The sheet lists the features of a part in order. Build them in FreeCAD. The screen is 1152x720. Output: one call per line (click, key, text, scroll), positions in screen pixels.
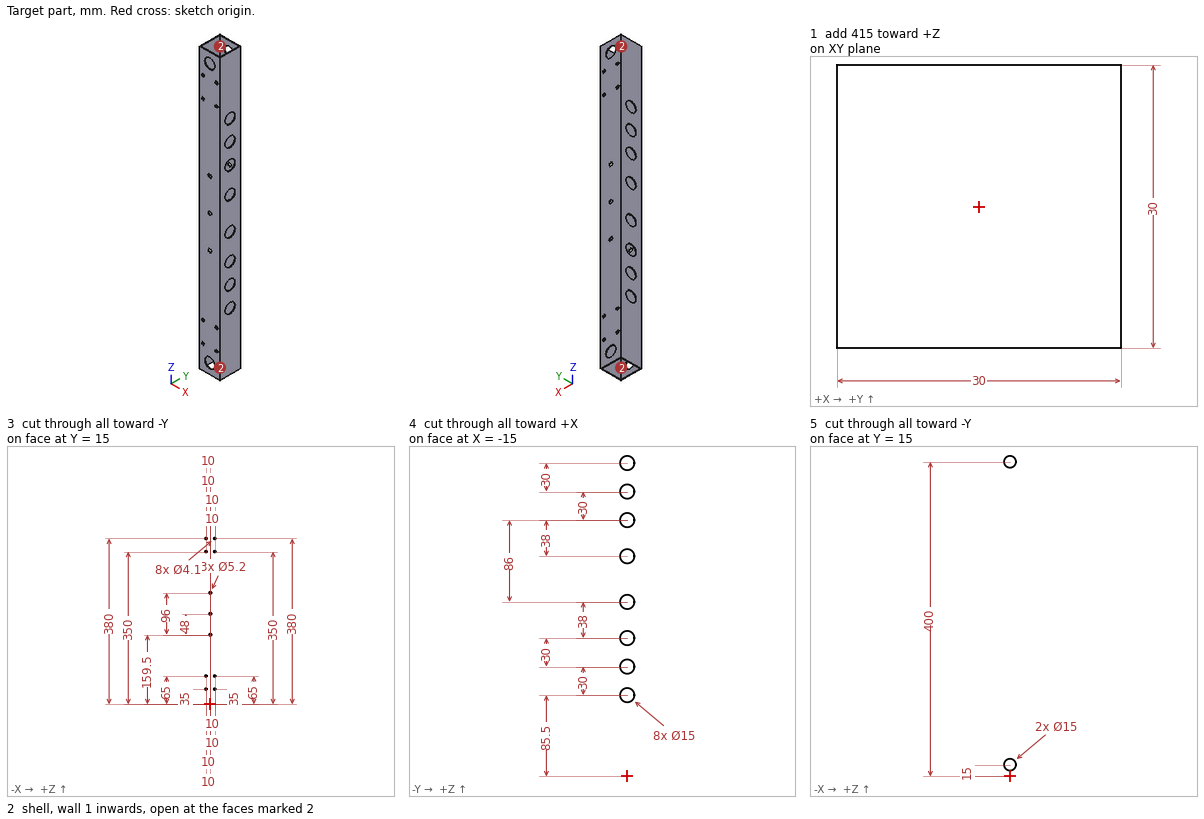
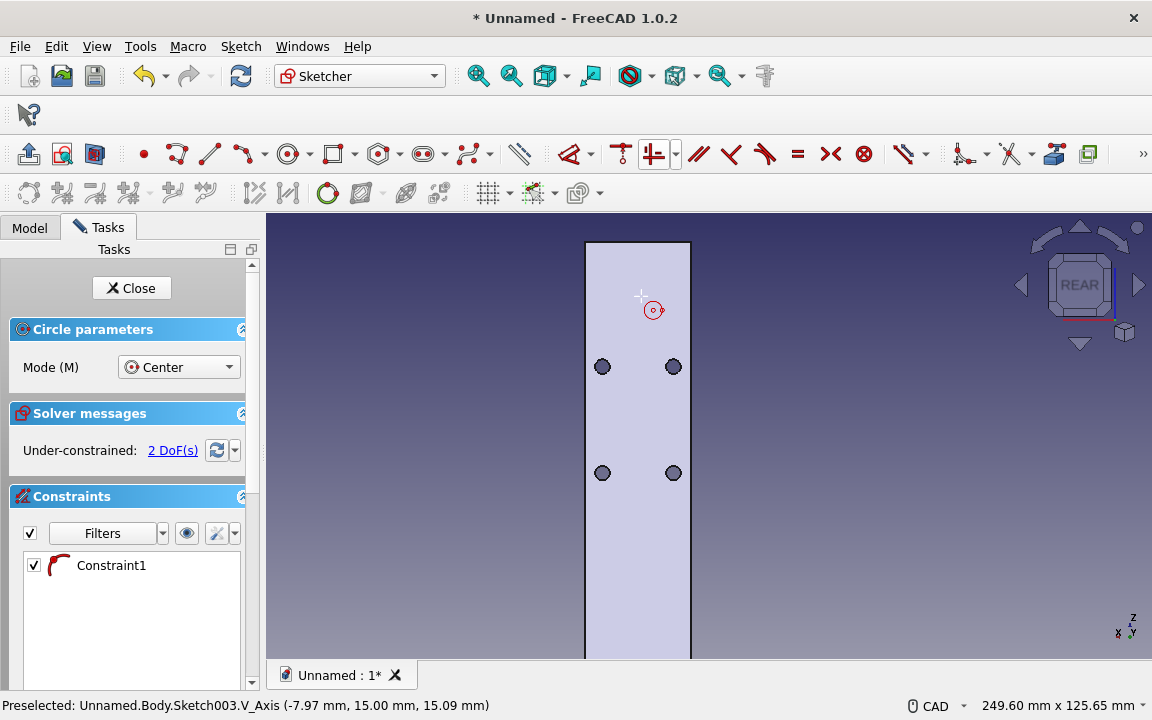
scroll(641, 295, down, 8)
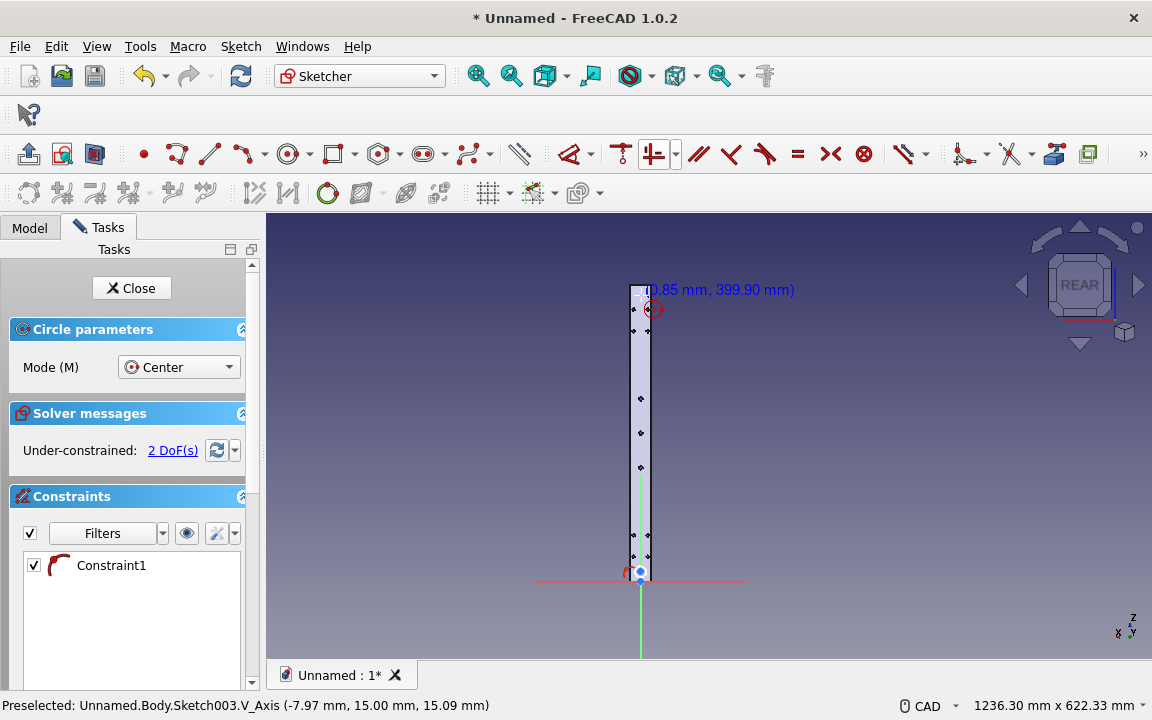
click(641, 295)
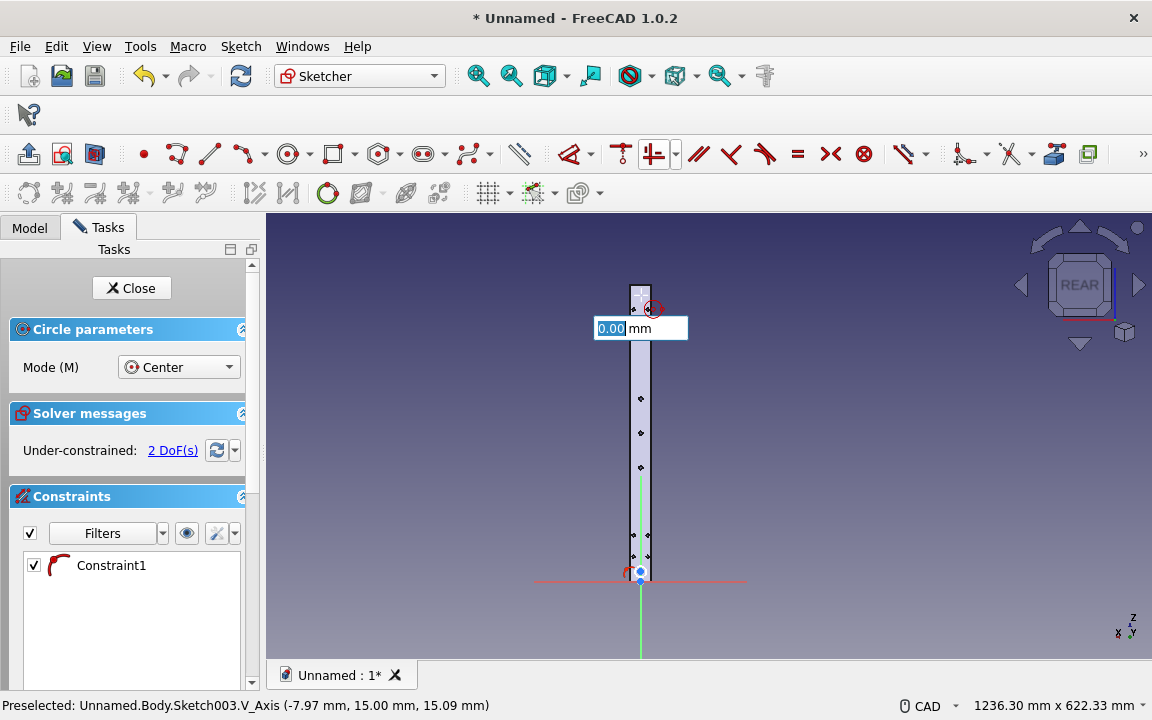
scroll(646, 293, up, 6)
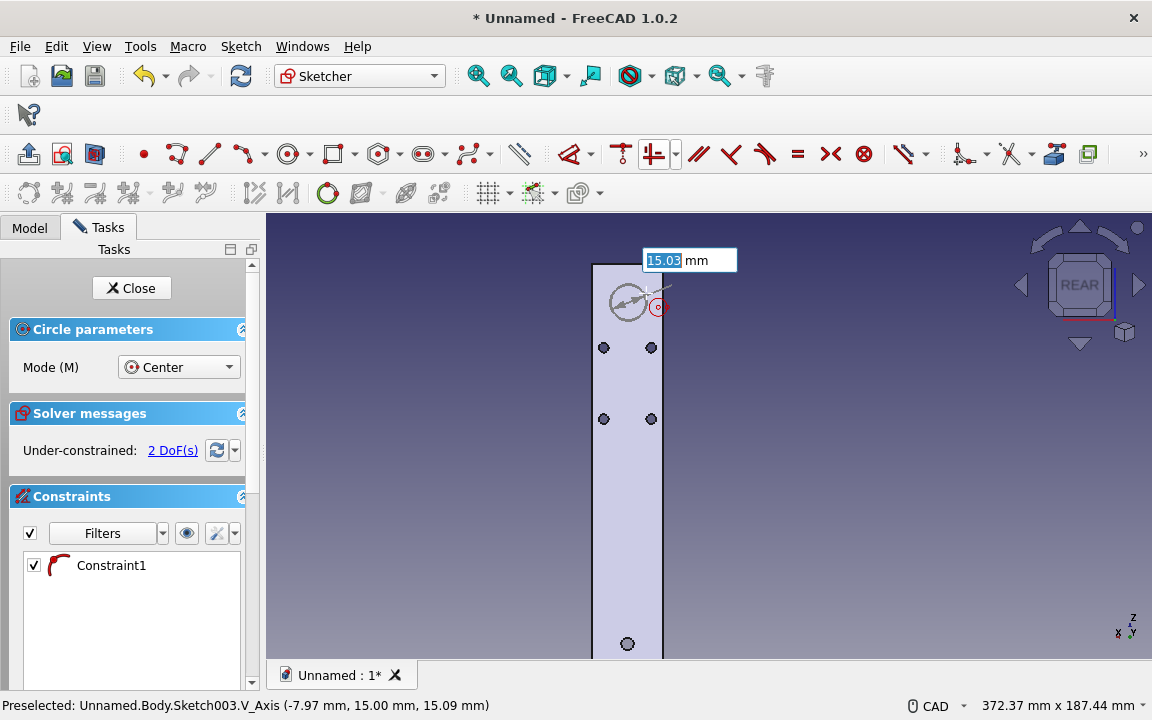
click(644, 294)
key(Escape)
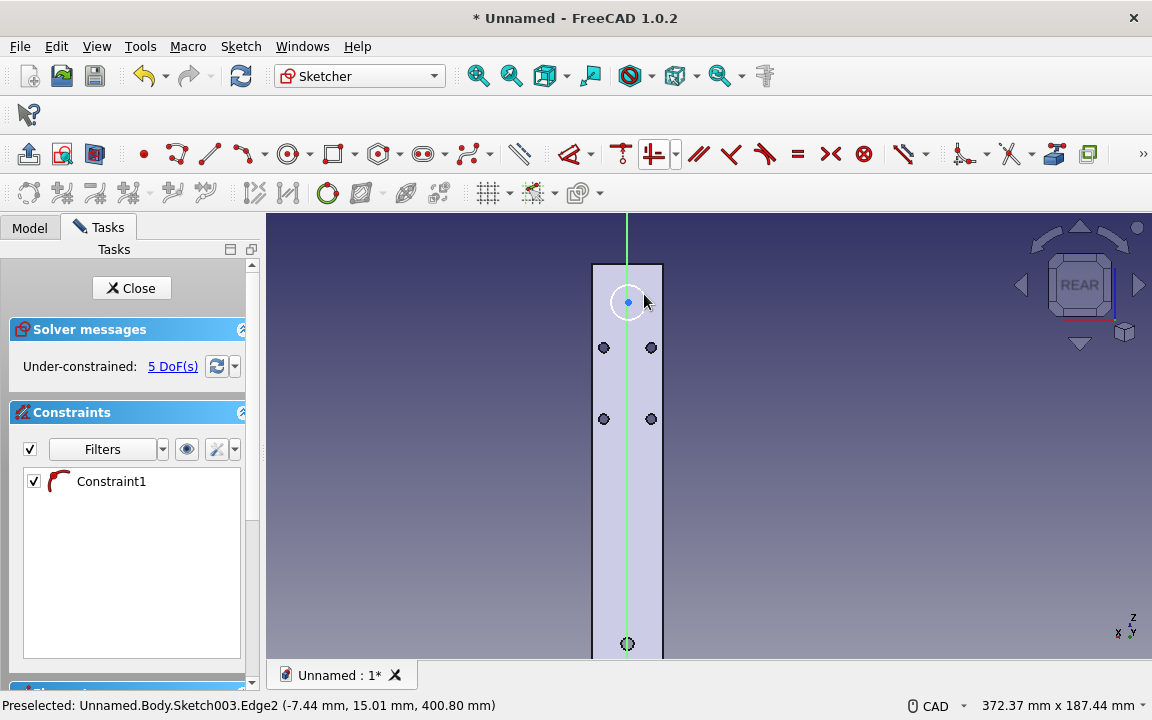
scroll(646, 293, down, 6)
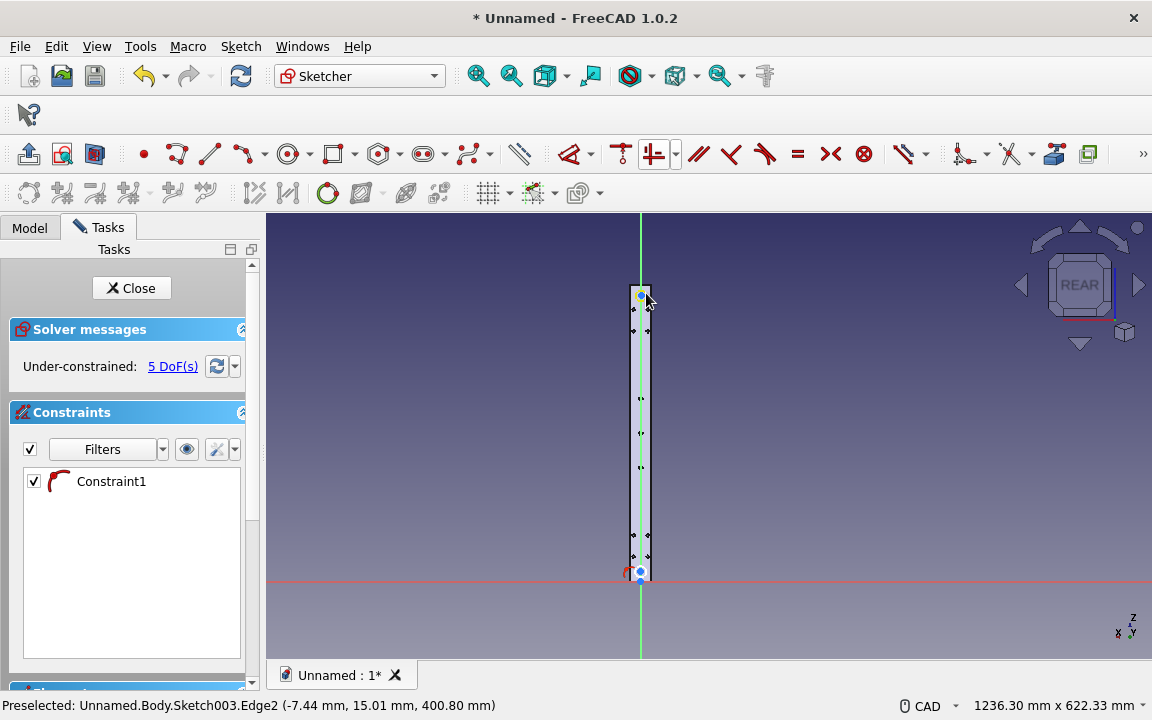
scroll(645, 568, up, 7)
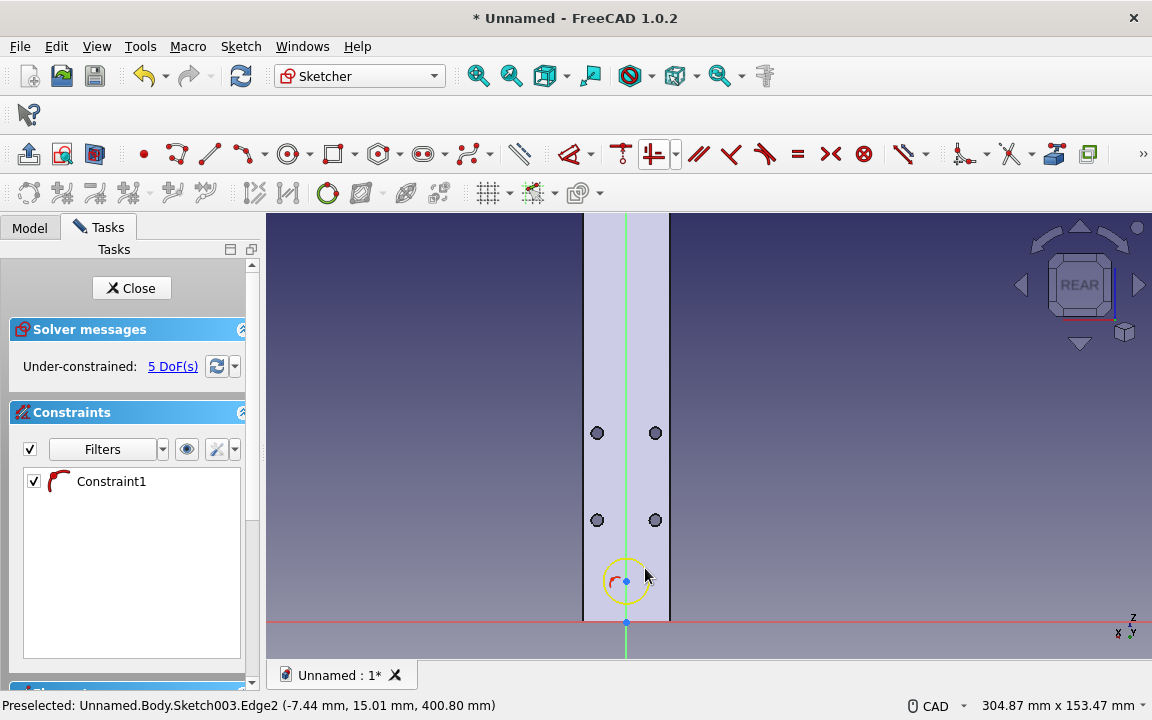
click(642, 565)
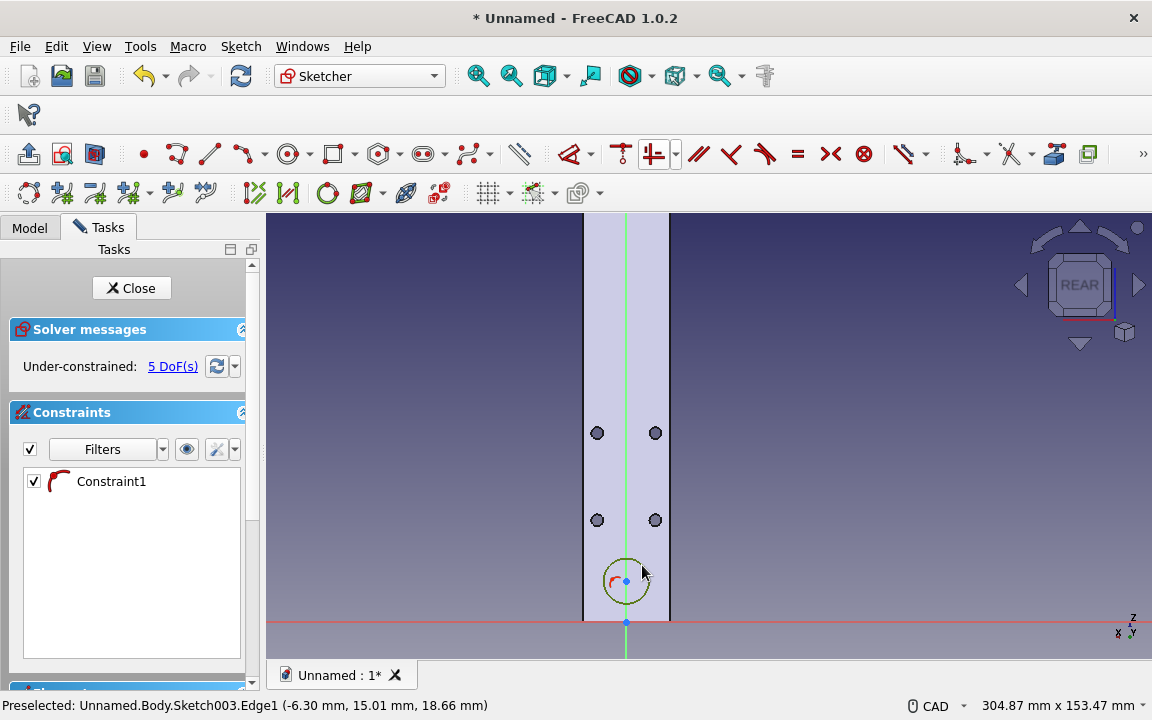
scroll(645, 569, down, 7)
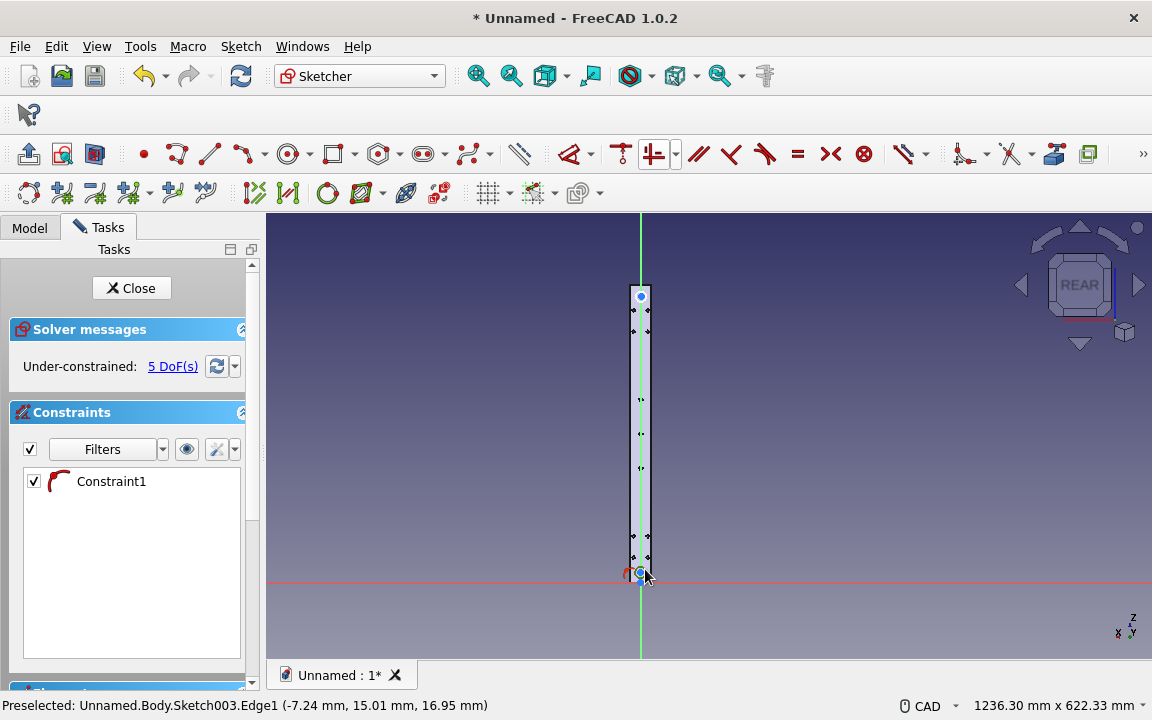
scroll(645, 293, up, 7)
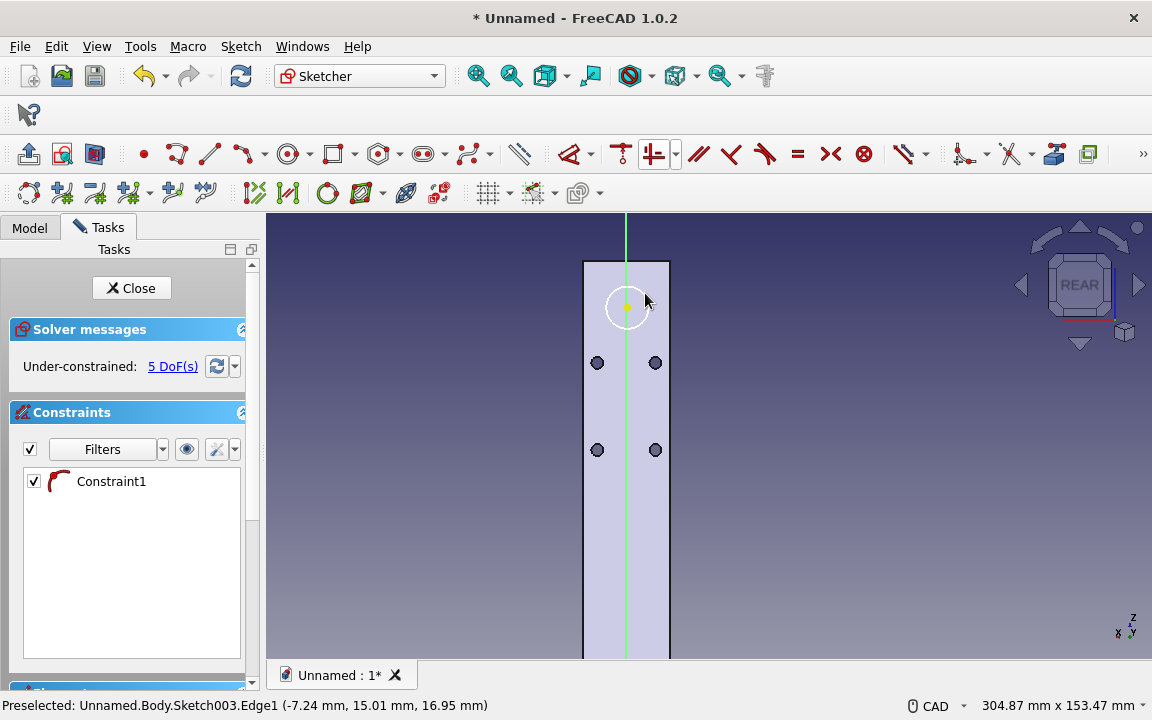
click(642, 293)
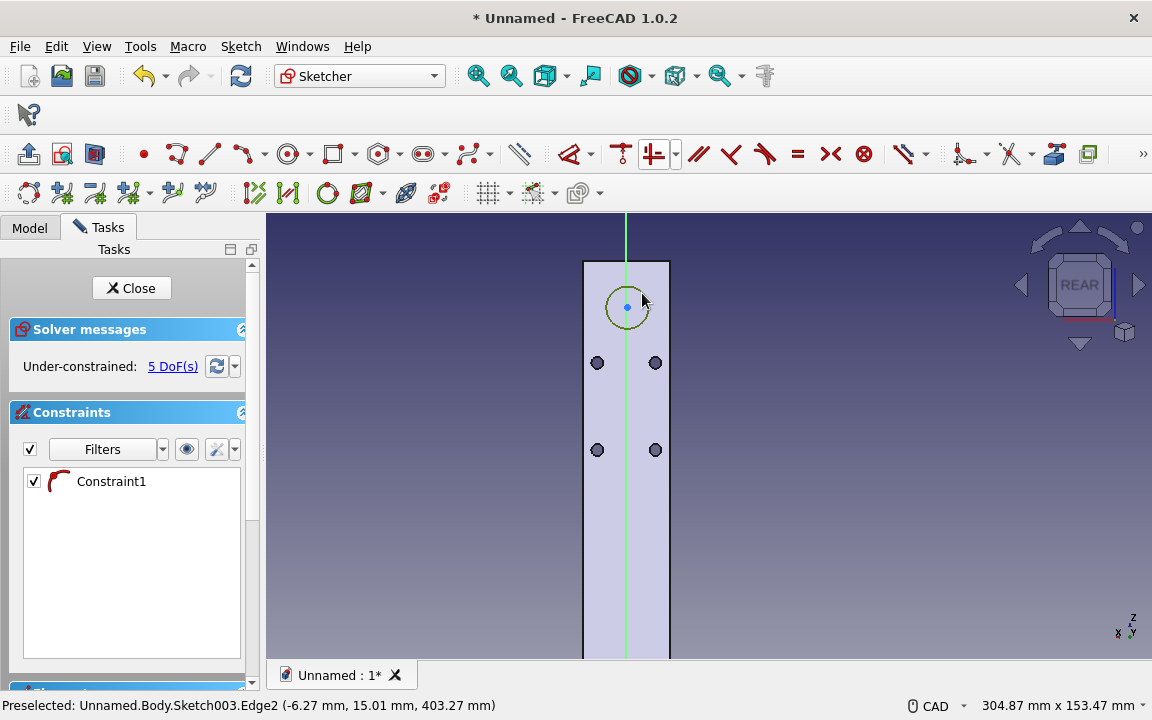
key(e)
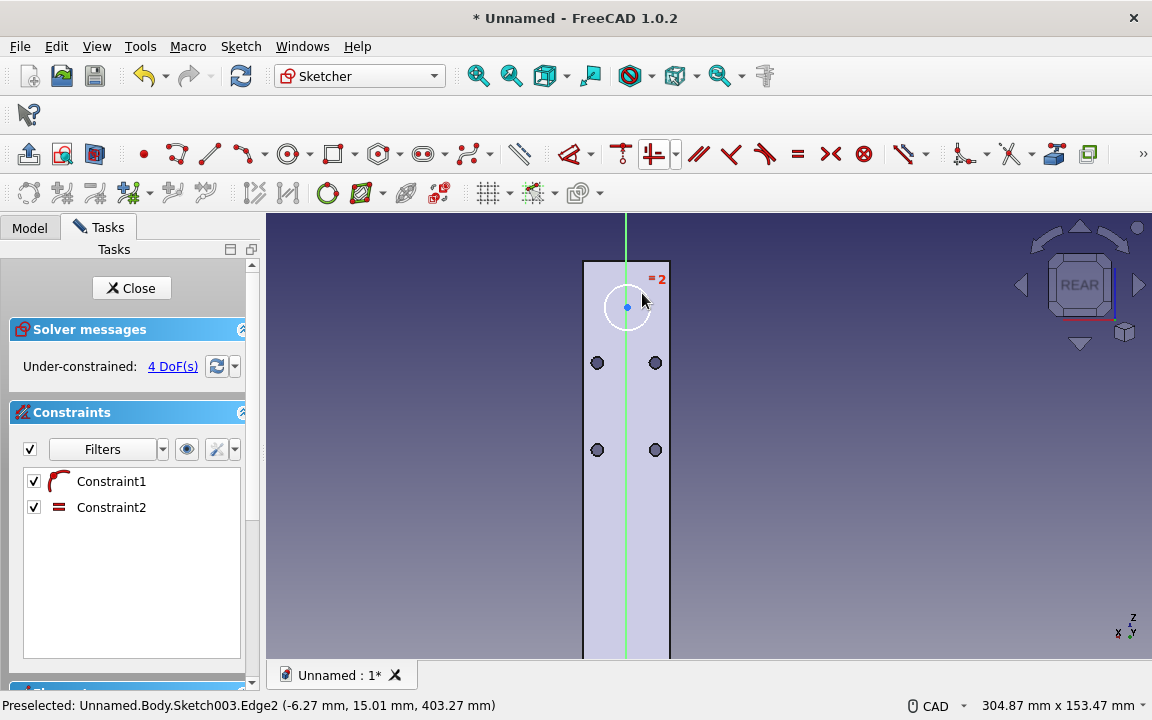
scroll(645, 292, down, 7)